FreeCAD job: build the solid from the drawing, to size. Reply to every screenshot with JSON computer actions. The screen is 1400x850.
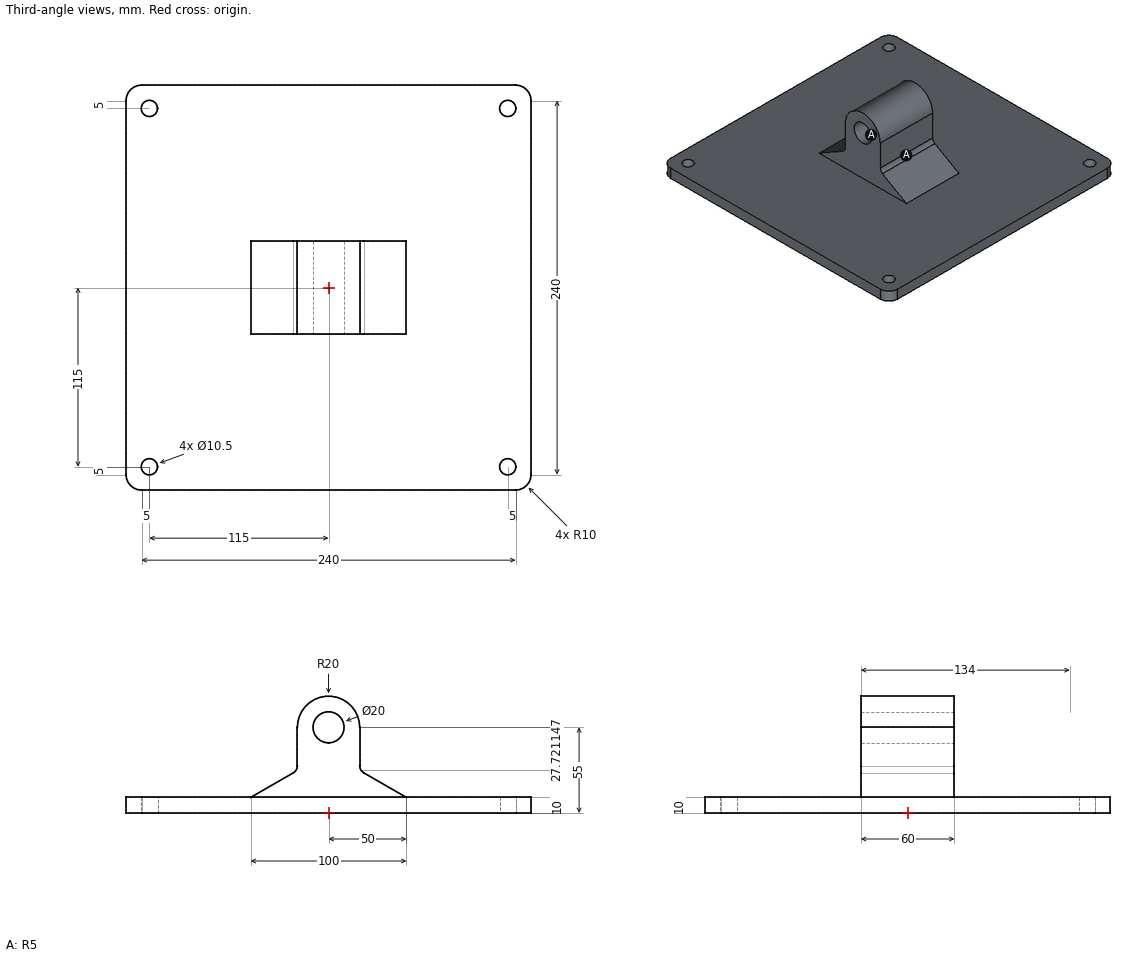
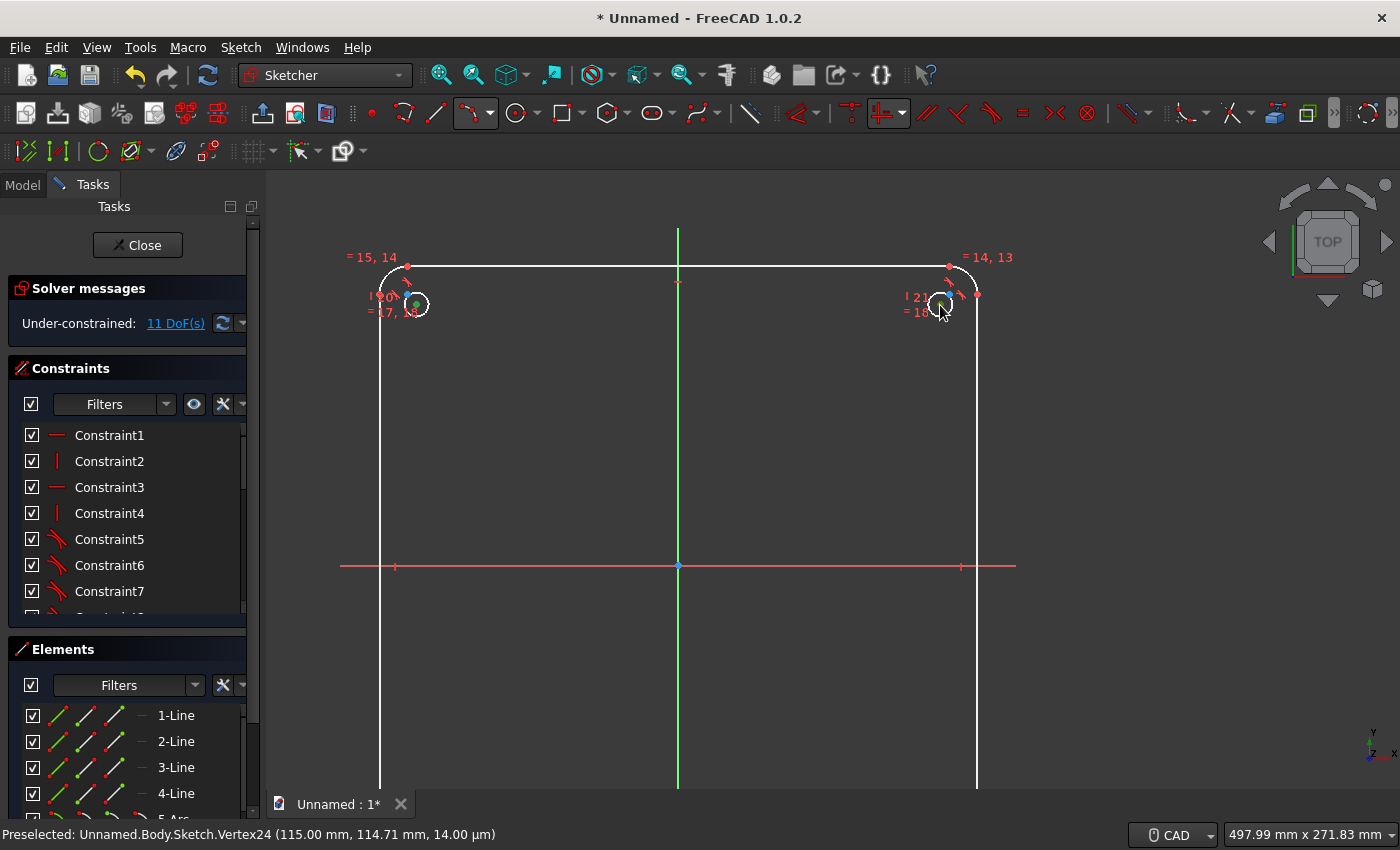
{"action": "key", "text": "h"}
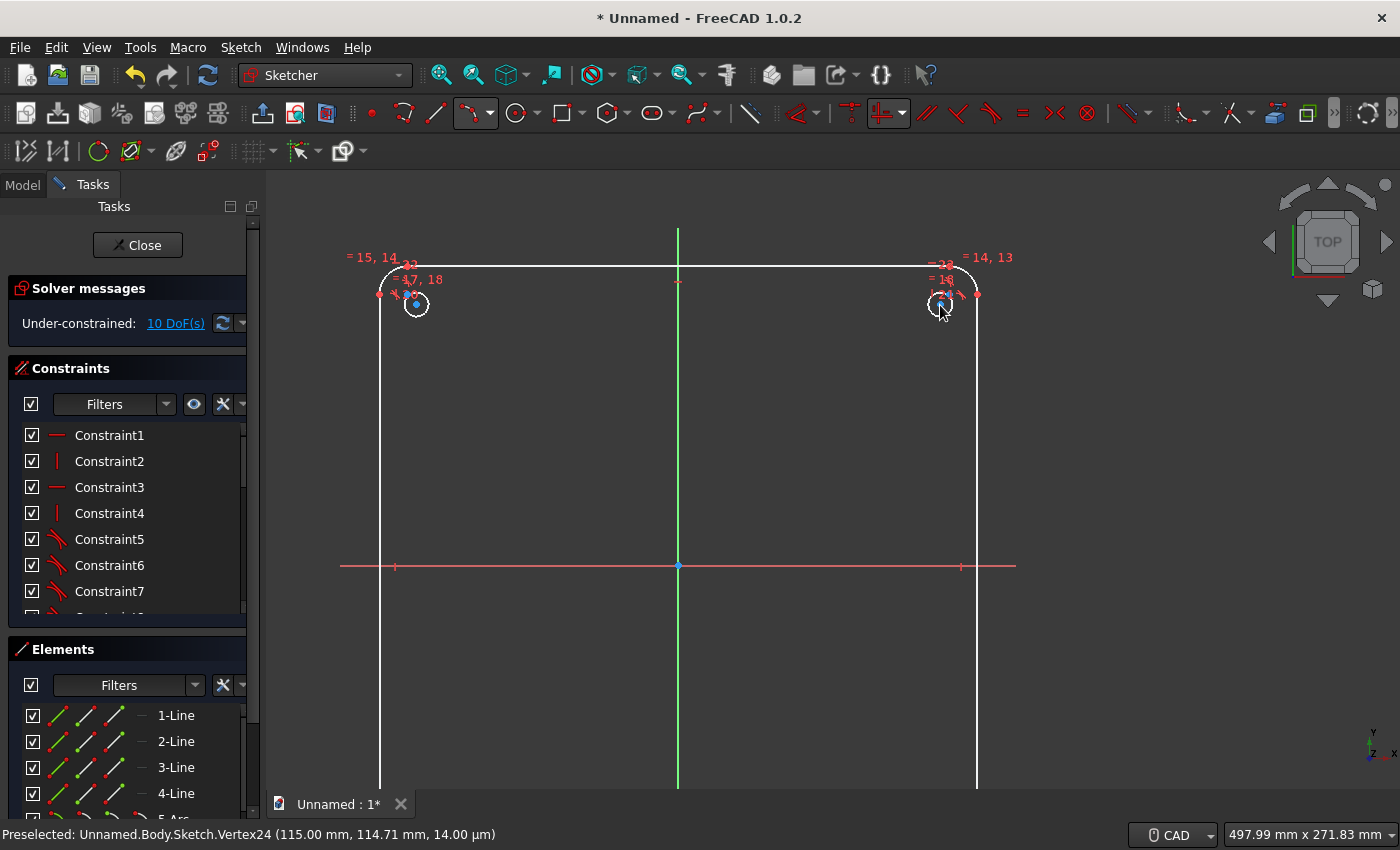
{"action": "left_click", "coordinate": [796, 114]}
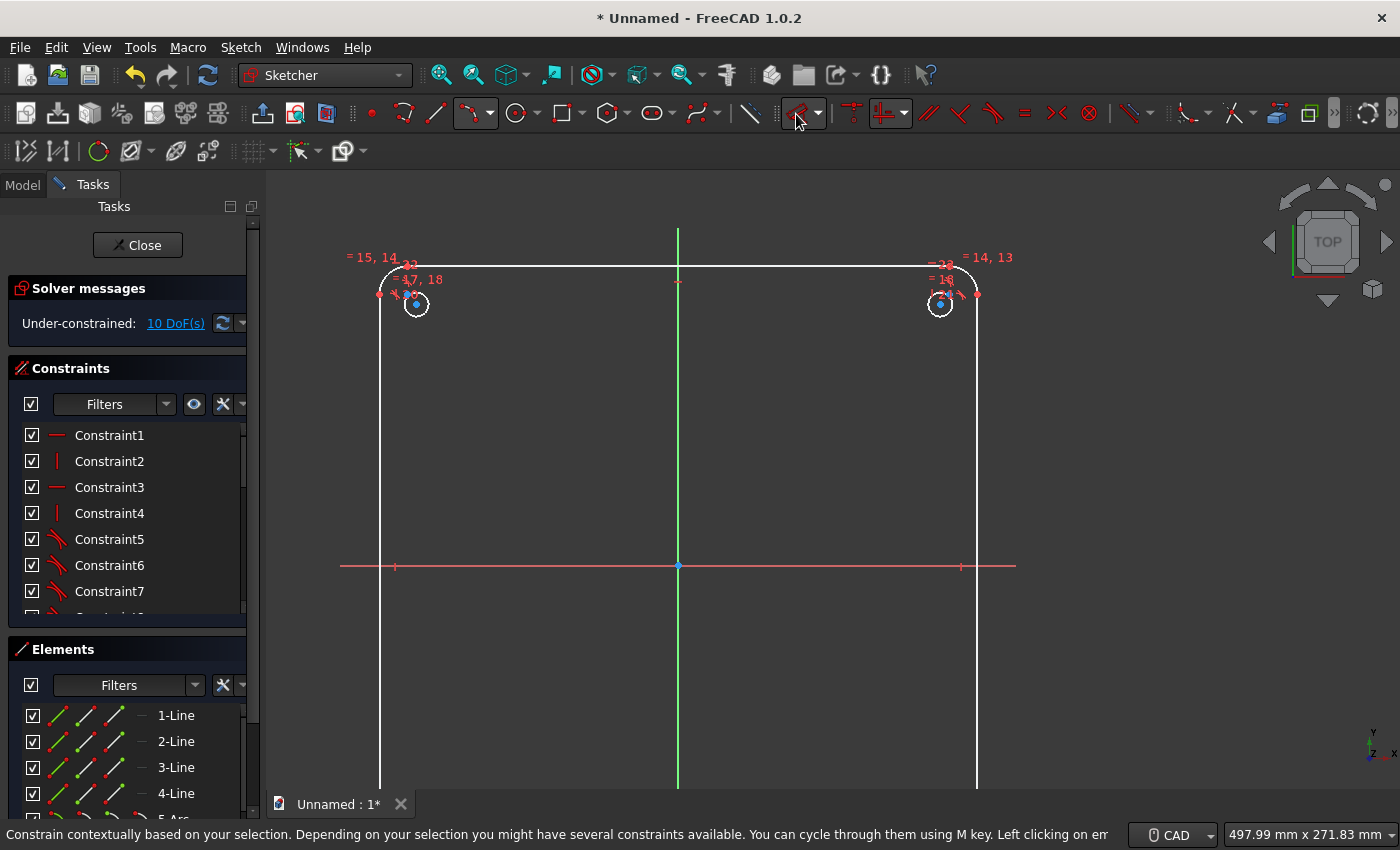
{"action": "scroll", "coordinate": [940, 304], "scroll_direction": "down", "scroll_amount": 2}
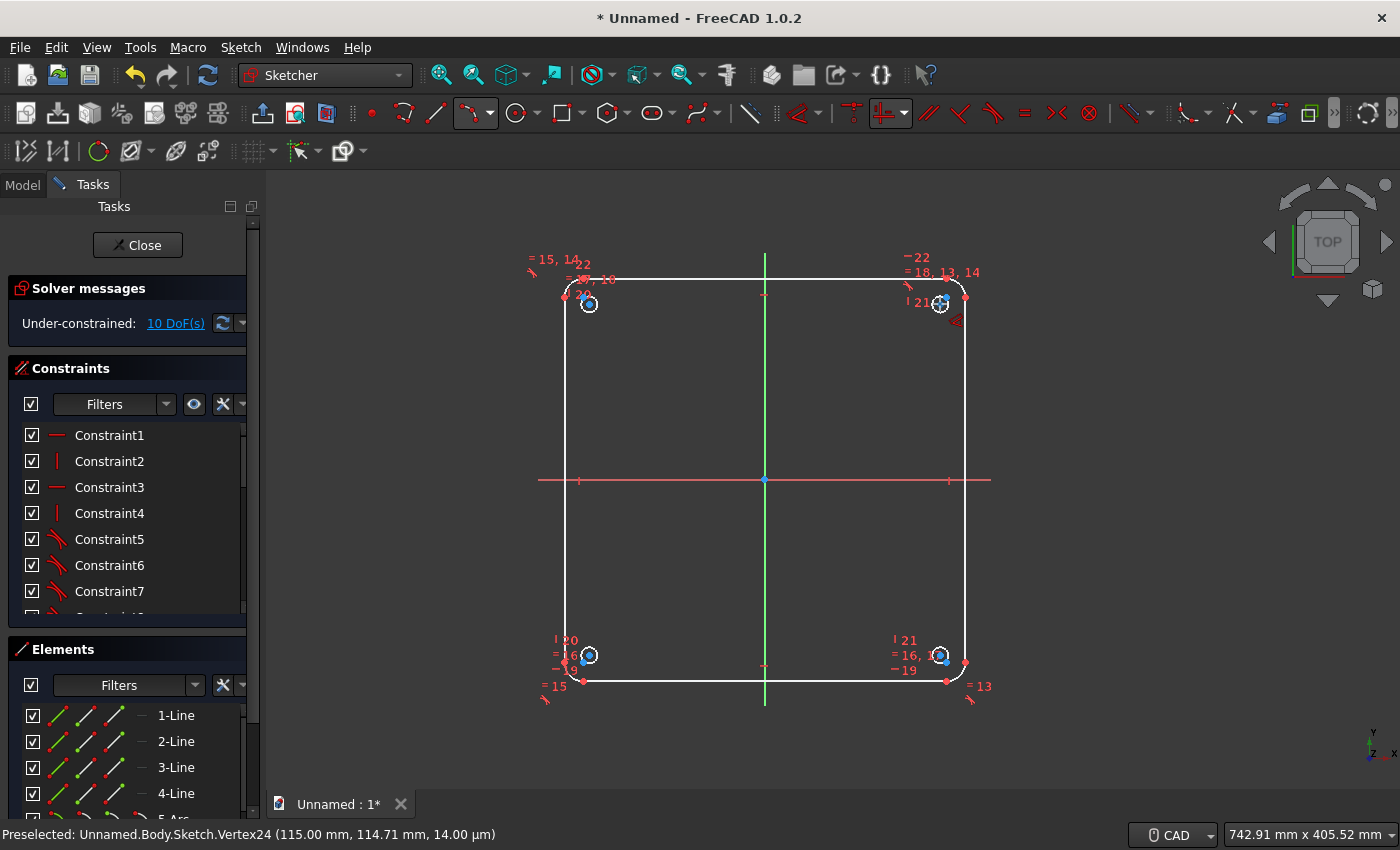
{"action": "scroll", "coordinate": [955, 679], "scroll_direction": "up", "scroll_amount": 5}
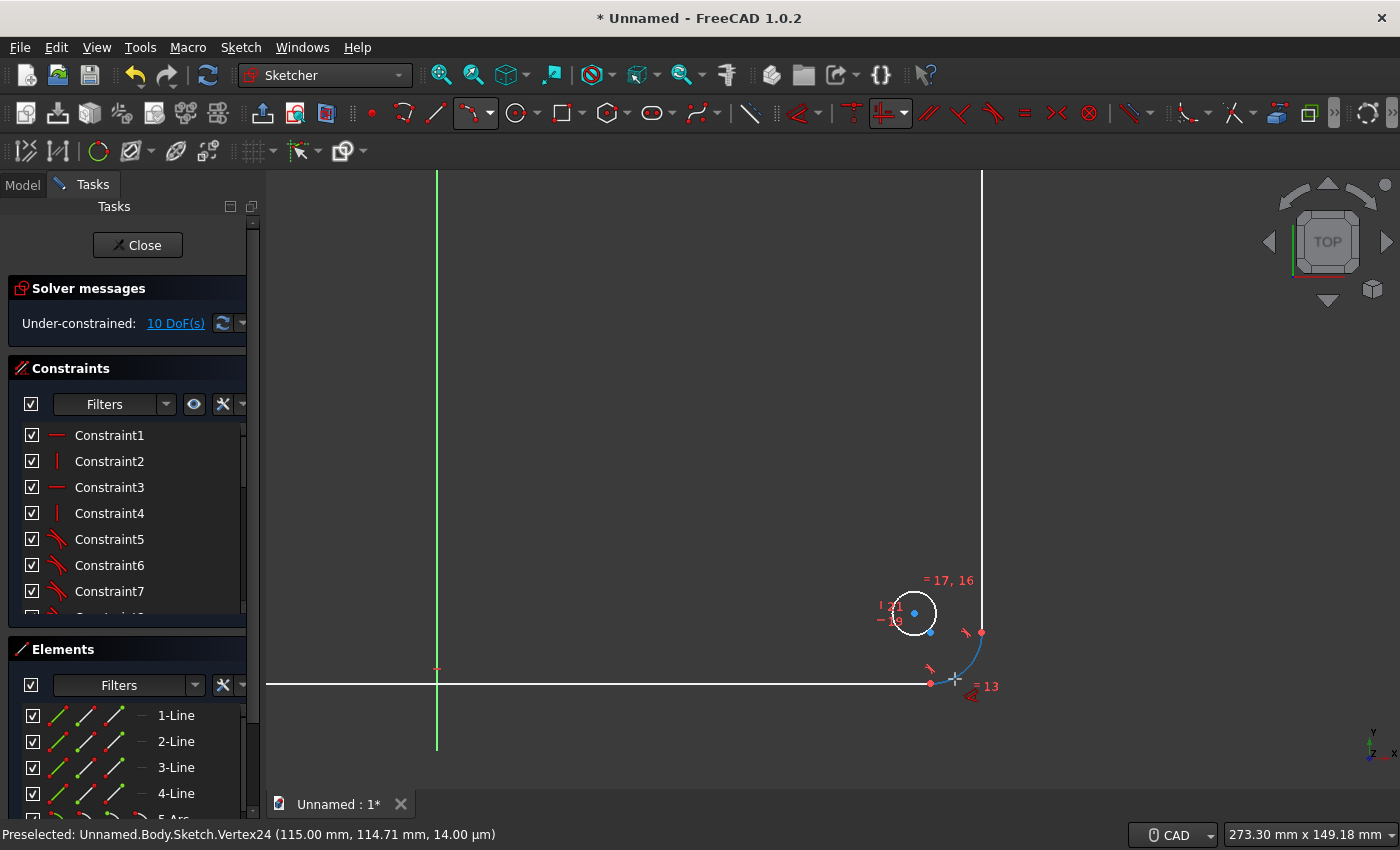
{"action": "left_click", "coordinate": [954, 678]}
{"action": "left_click", "coordinate": [969, 706]}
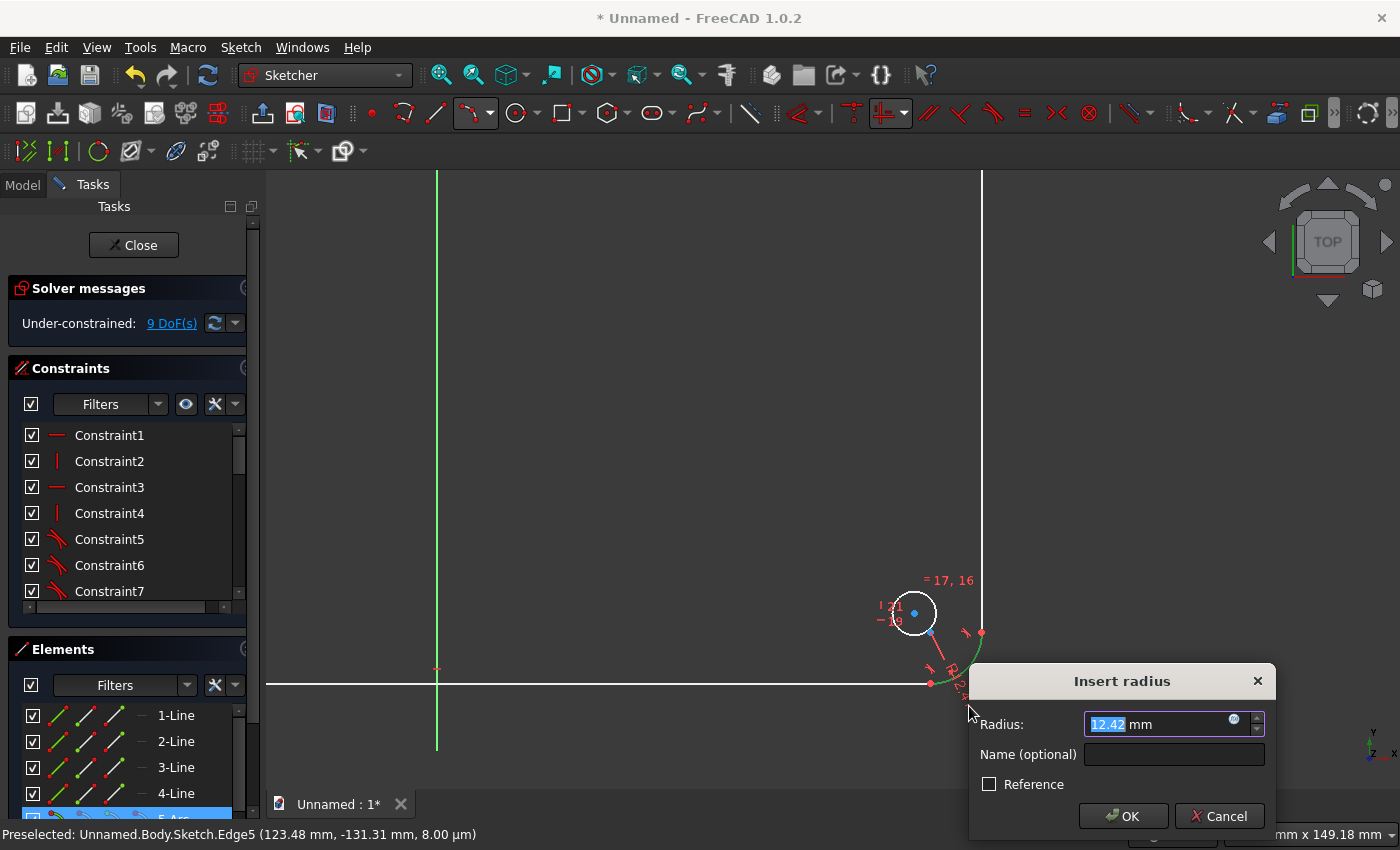
{"action": "type", "text": "10"}
{"action": "key", "text": "Return"}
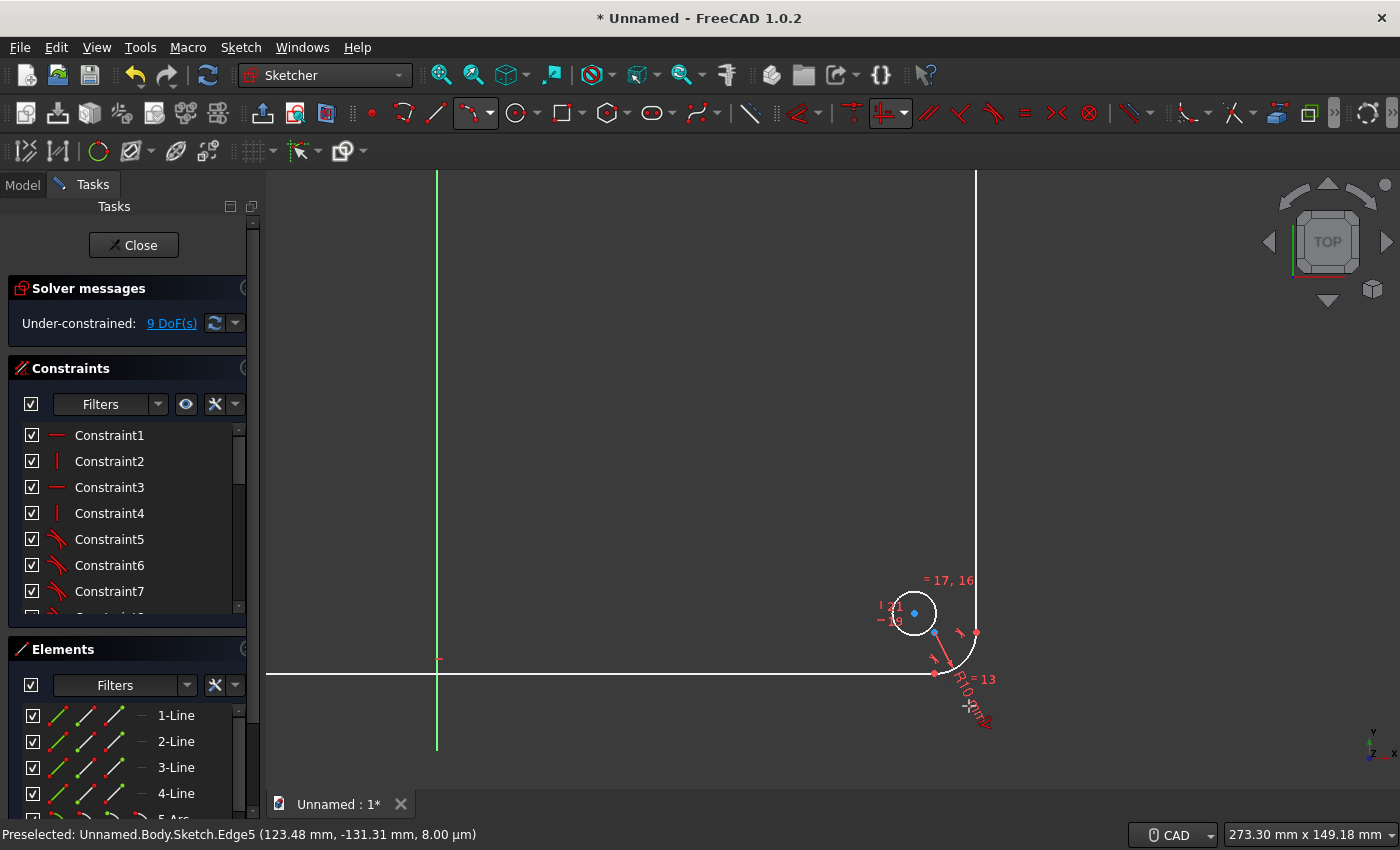
{"action": "scroll", "coordinate": [955, 680], "scroll_direction": "down", "scroll_amount": 5}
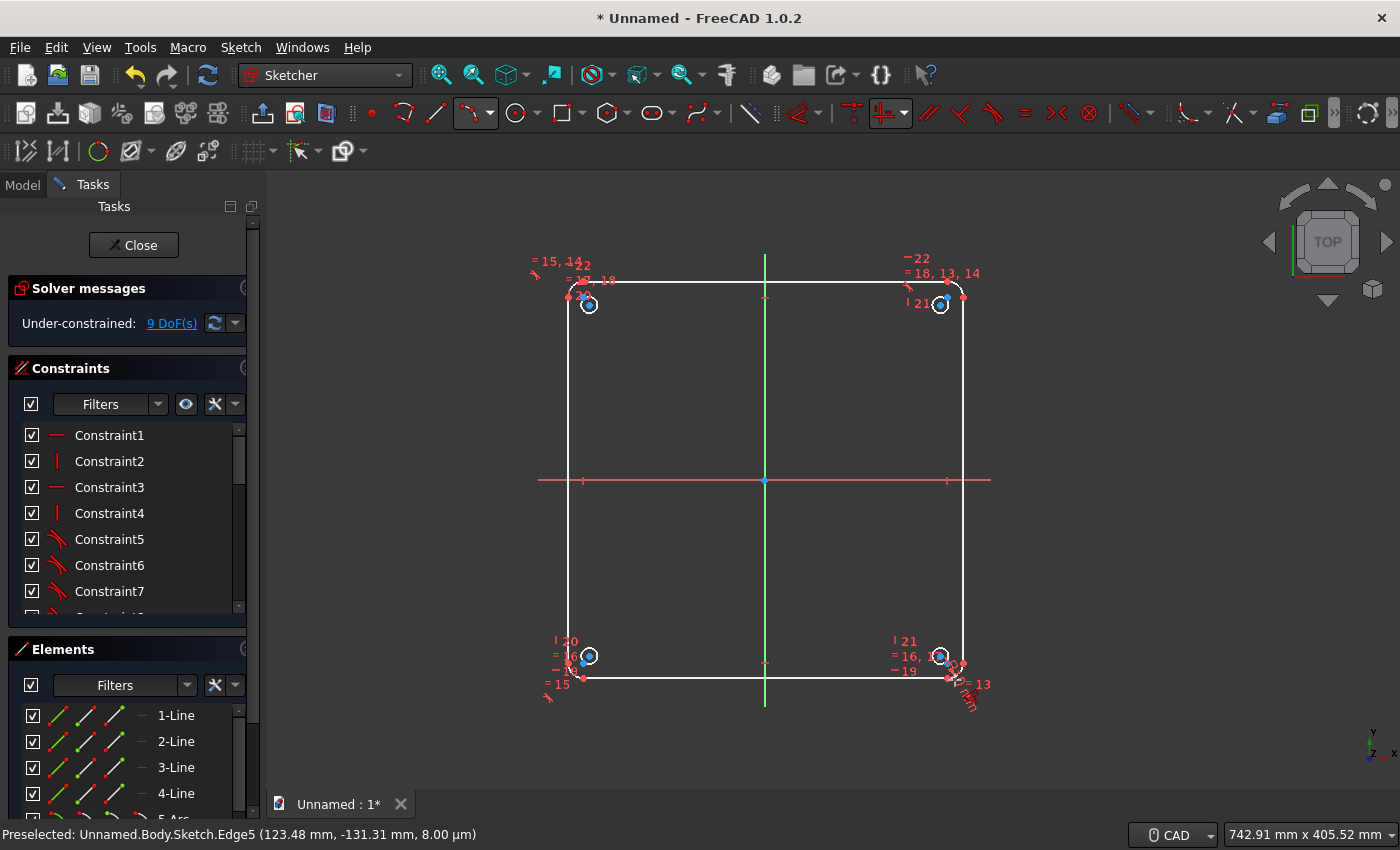
{"action": "scroll", "coordinate": [595, 650], "scroll_direction": "up", "scroll_amount": 5}